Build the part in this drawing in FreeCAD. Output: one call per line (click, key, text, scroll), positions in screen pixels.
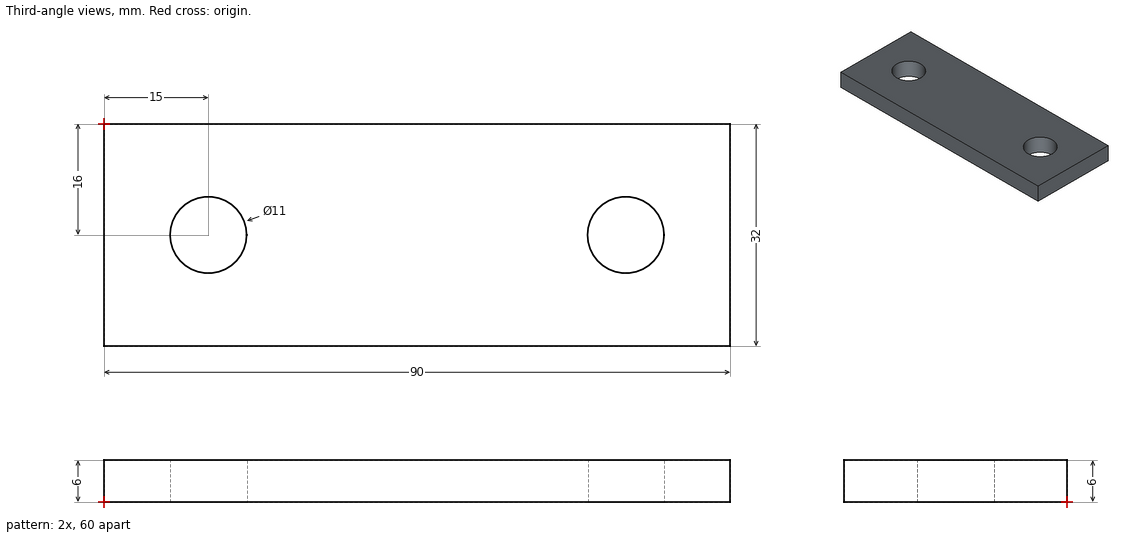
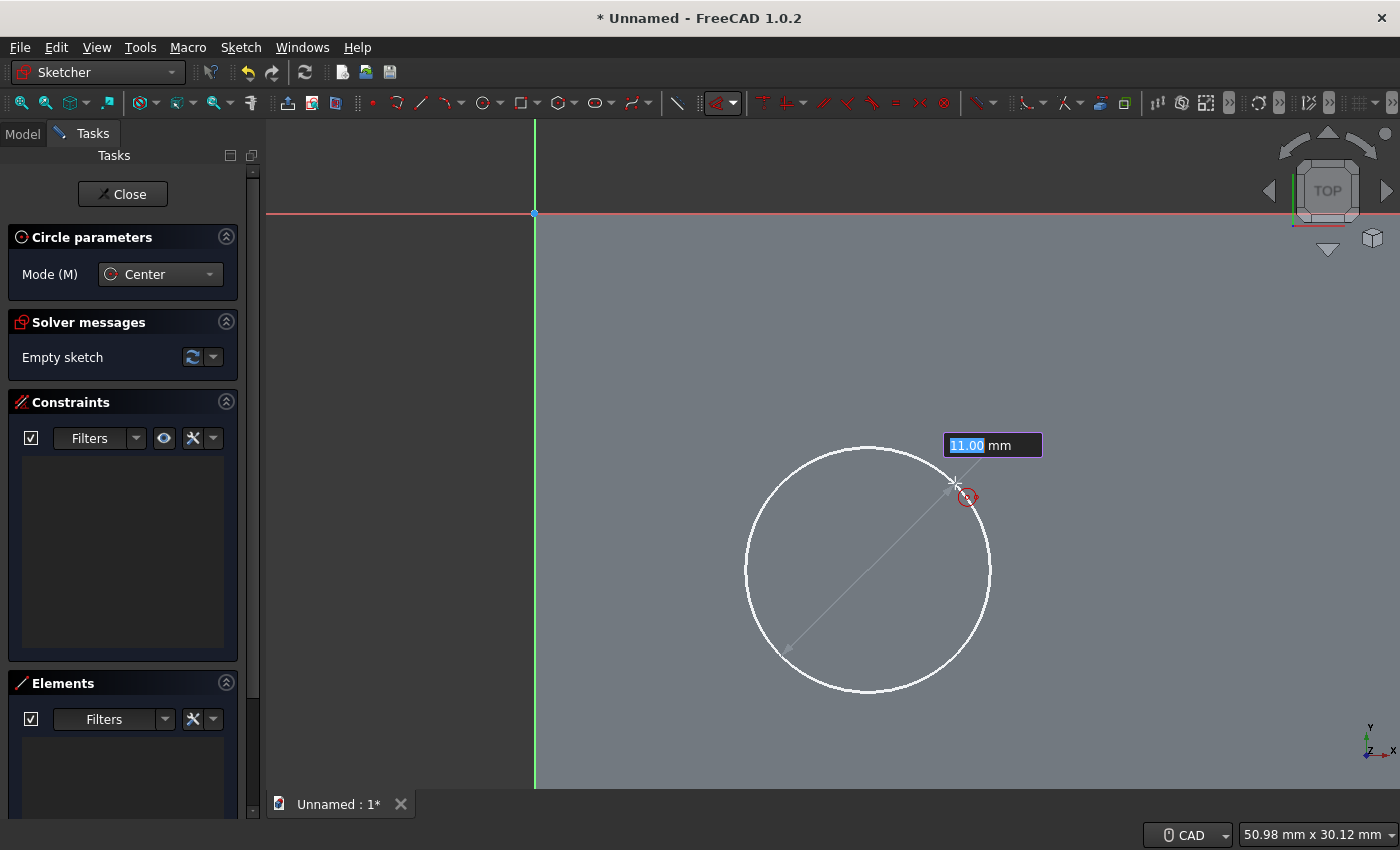
text(11)
key(Return)
key(Escape)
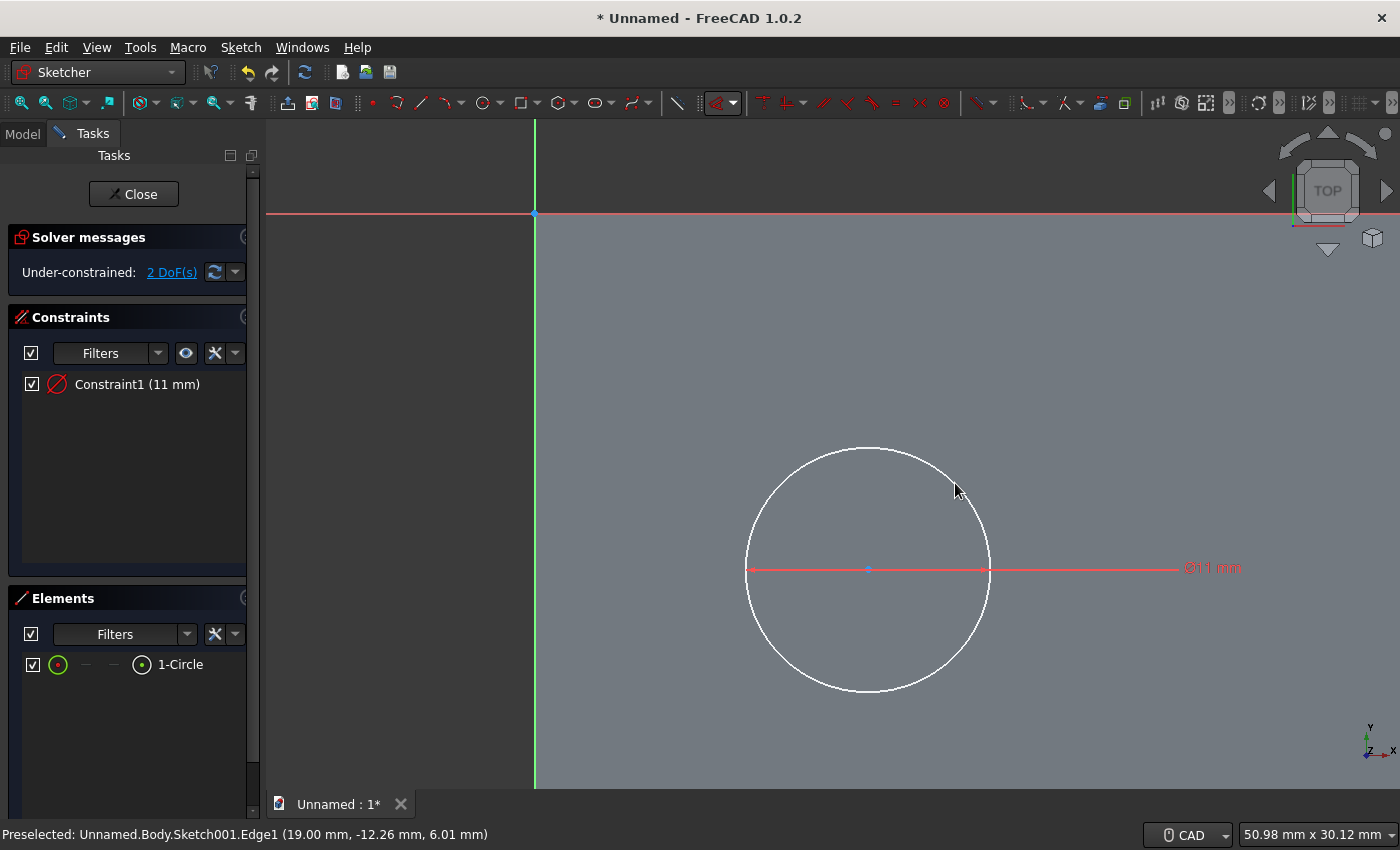
click(716, 104)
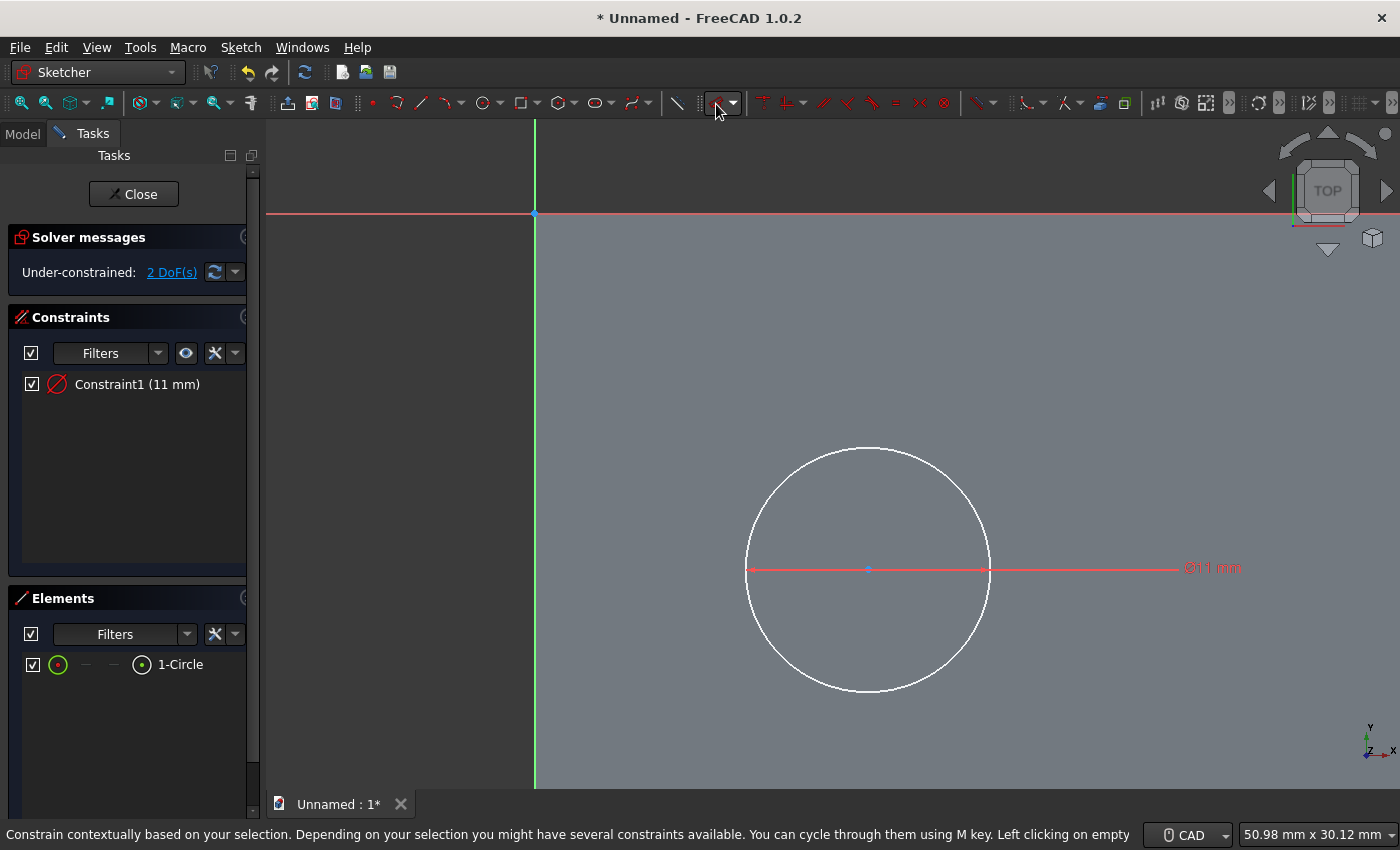
click(868, 570)
click(701, 180)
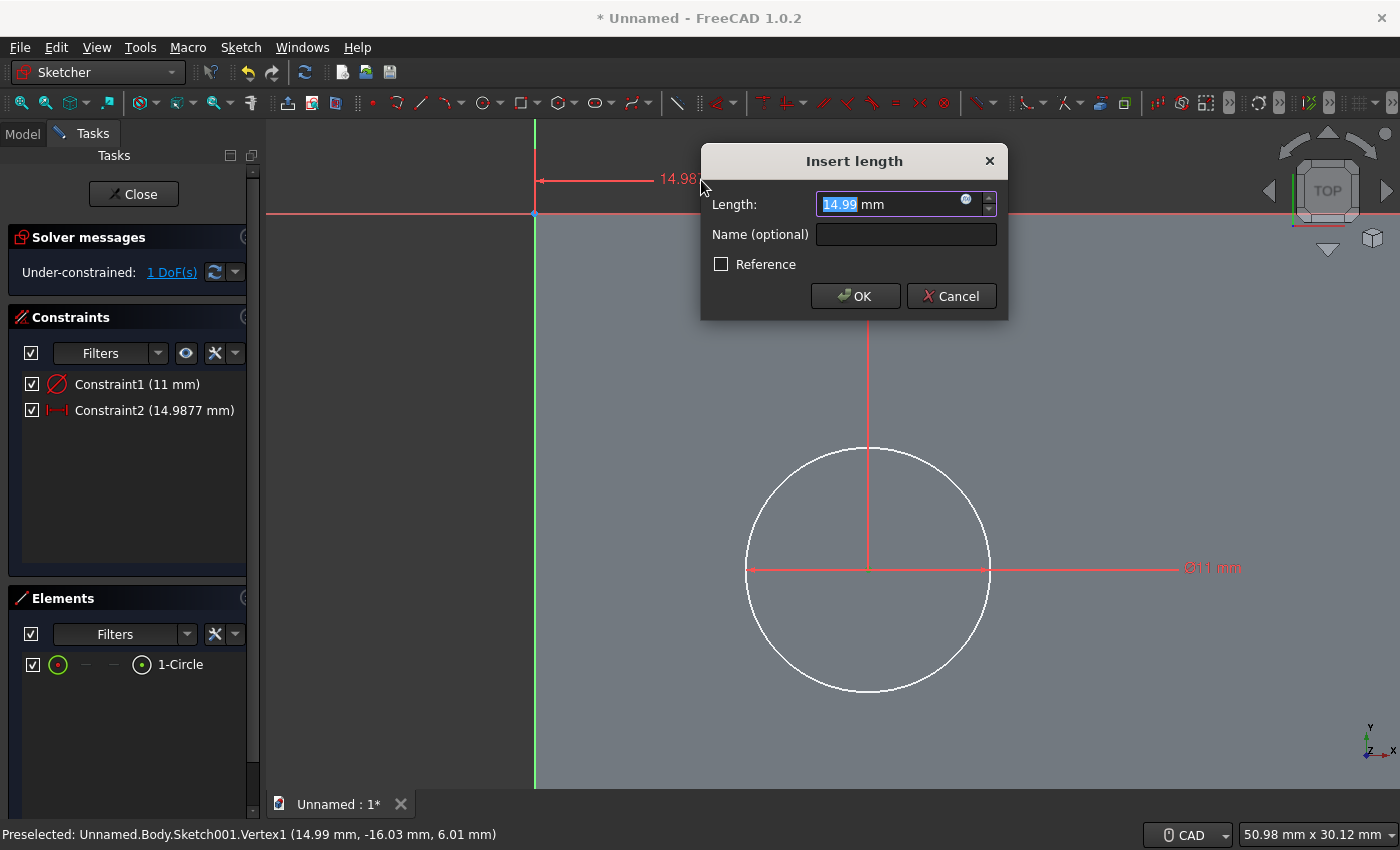
text(15)
key(Return)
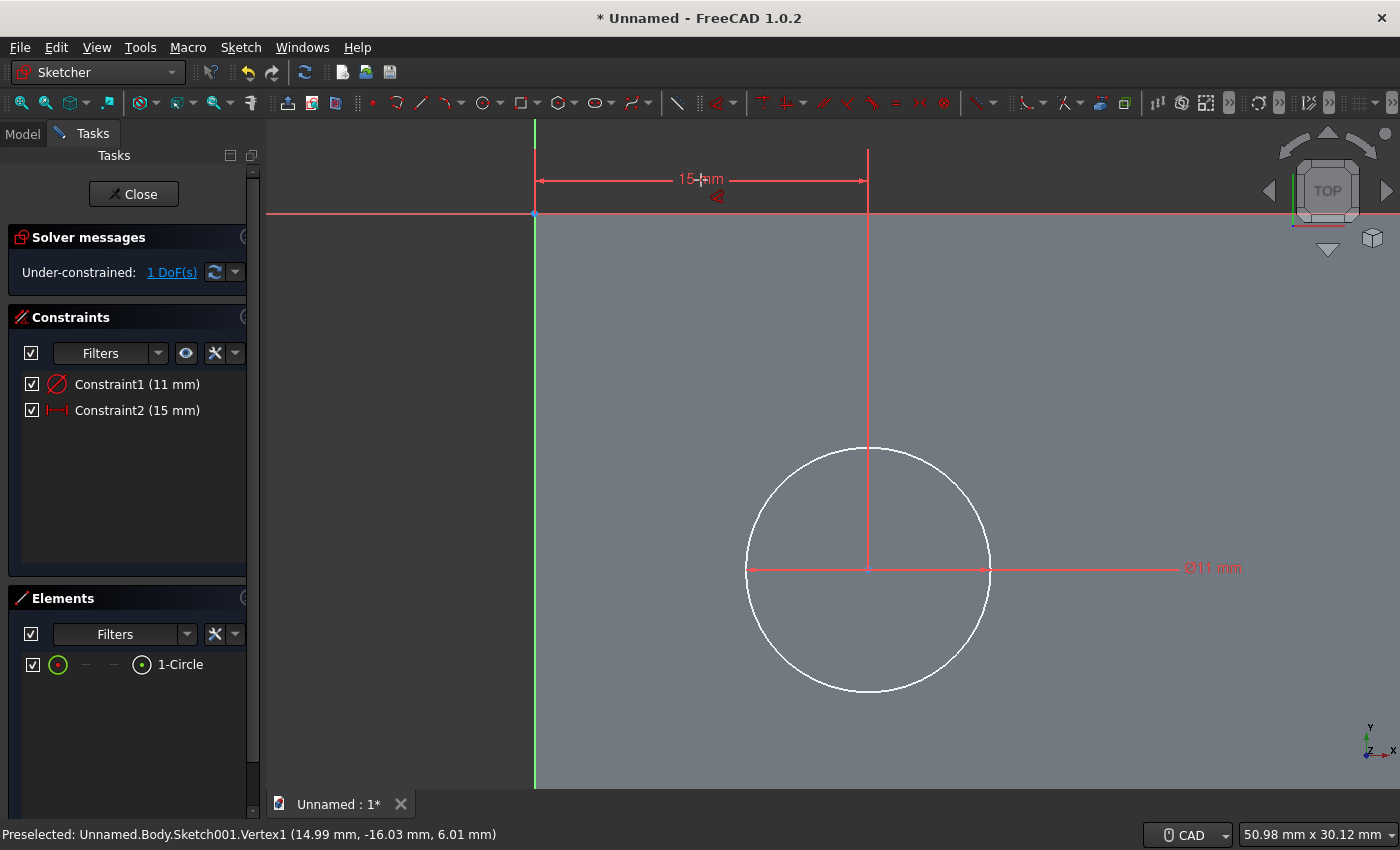
click(868, 570)
click(501, 392)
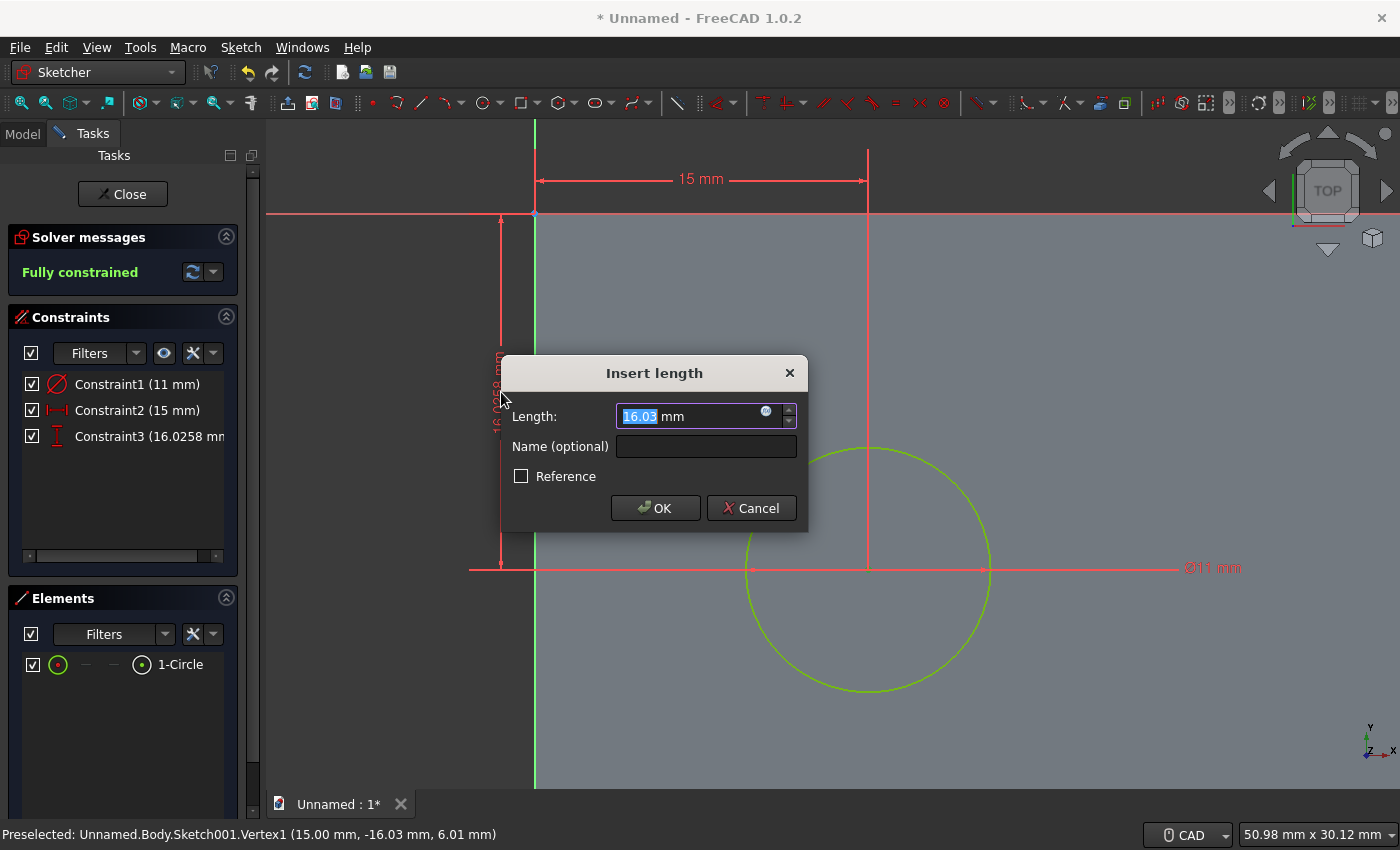
text(16)
key(Return)
key(Escape)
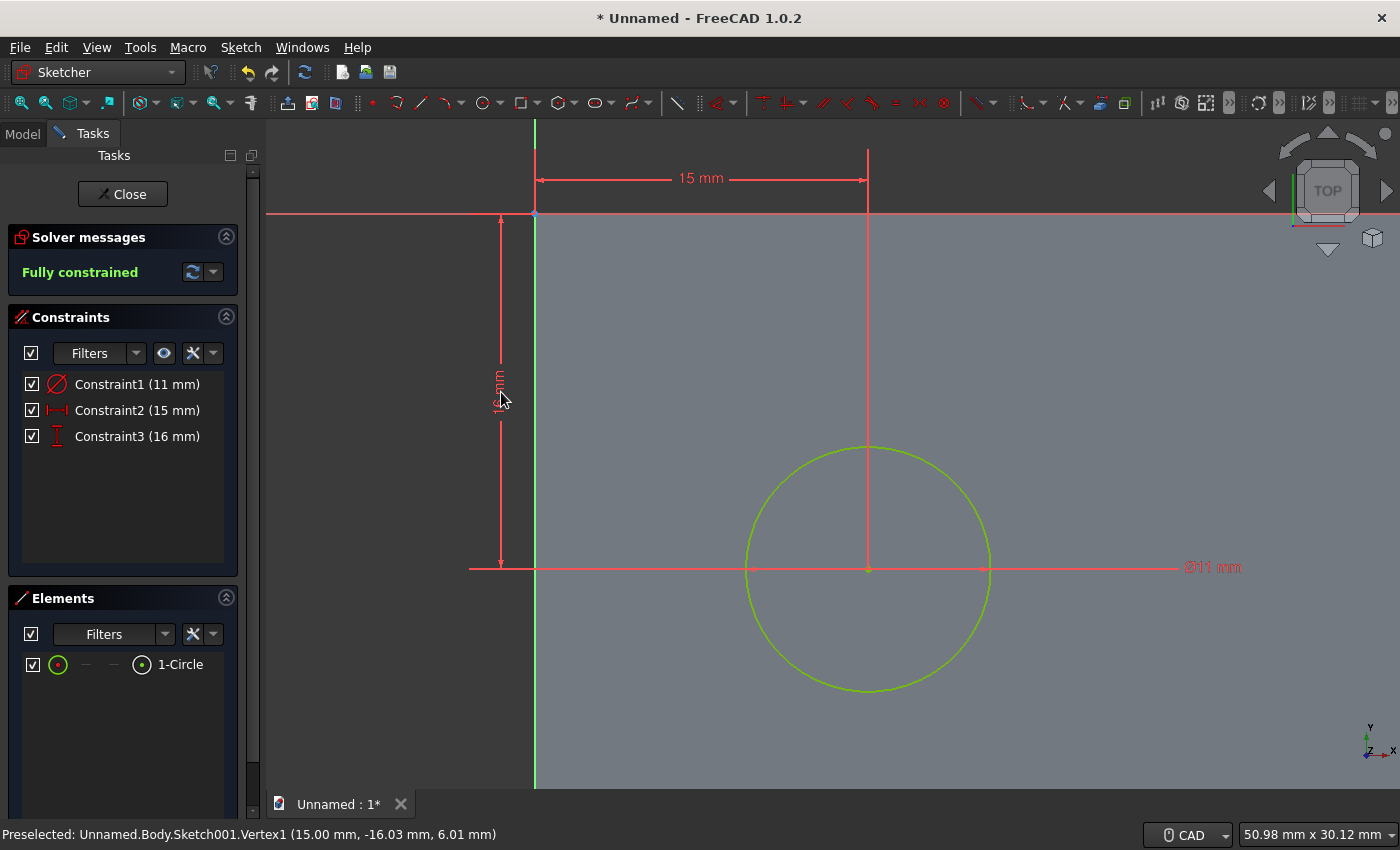
click(123, 194)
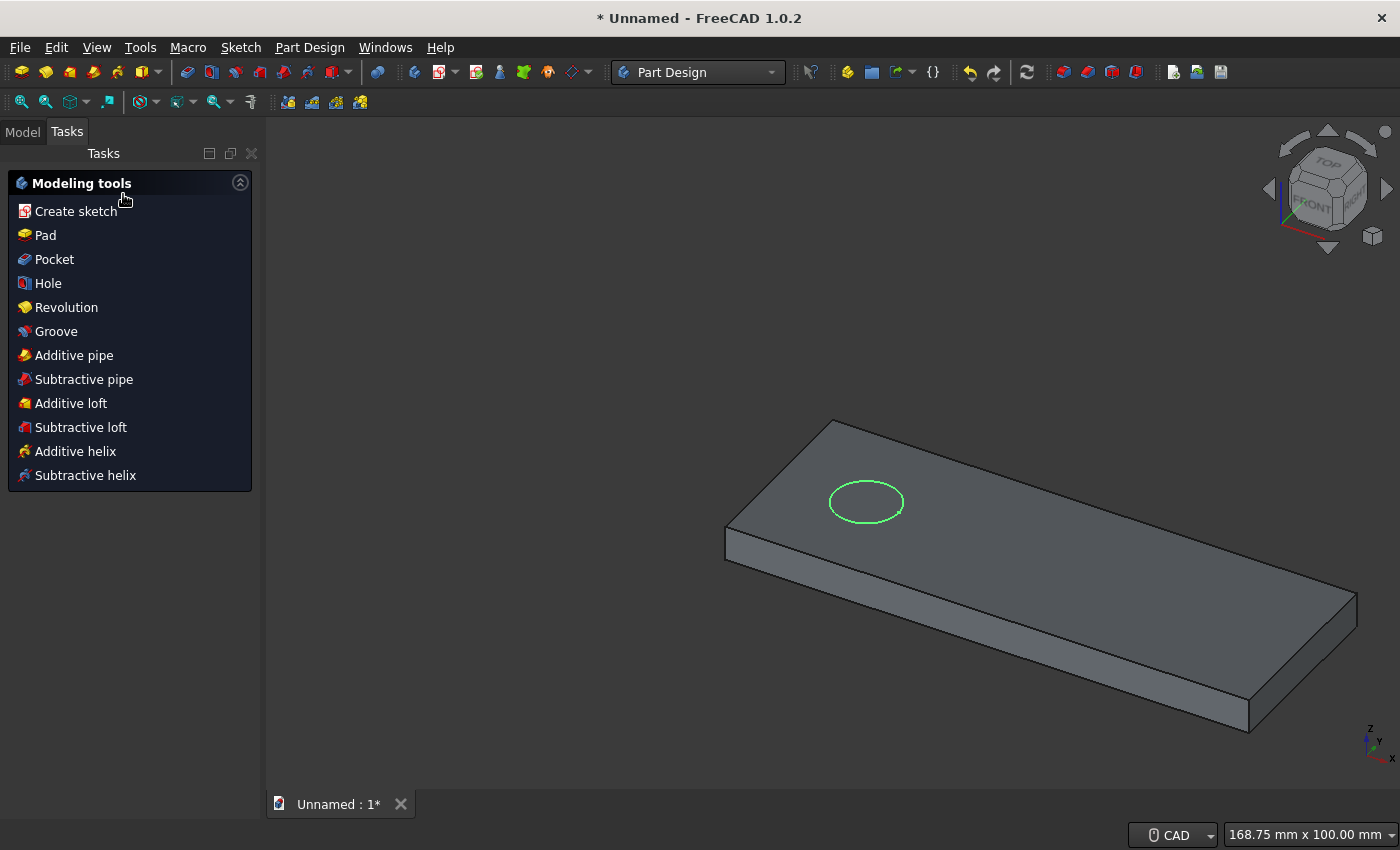
click(188, 72)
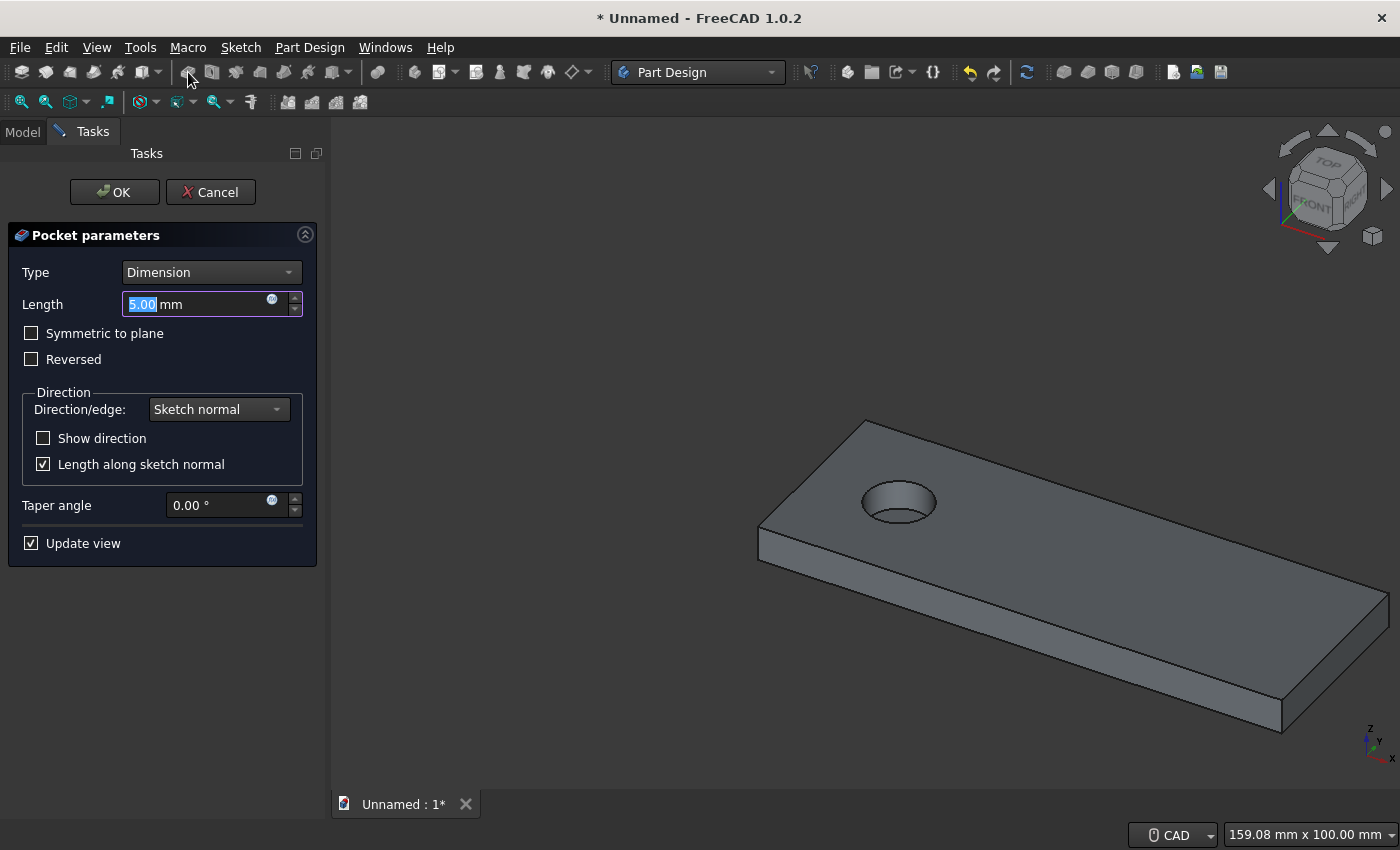
text(6)
key(Tab)